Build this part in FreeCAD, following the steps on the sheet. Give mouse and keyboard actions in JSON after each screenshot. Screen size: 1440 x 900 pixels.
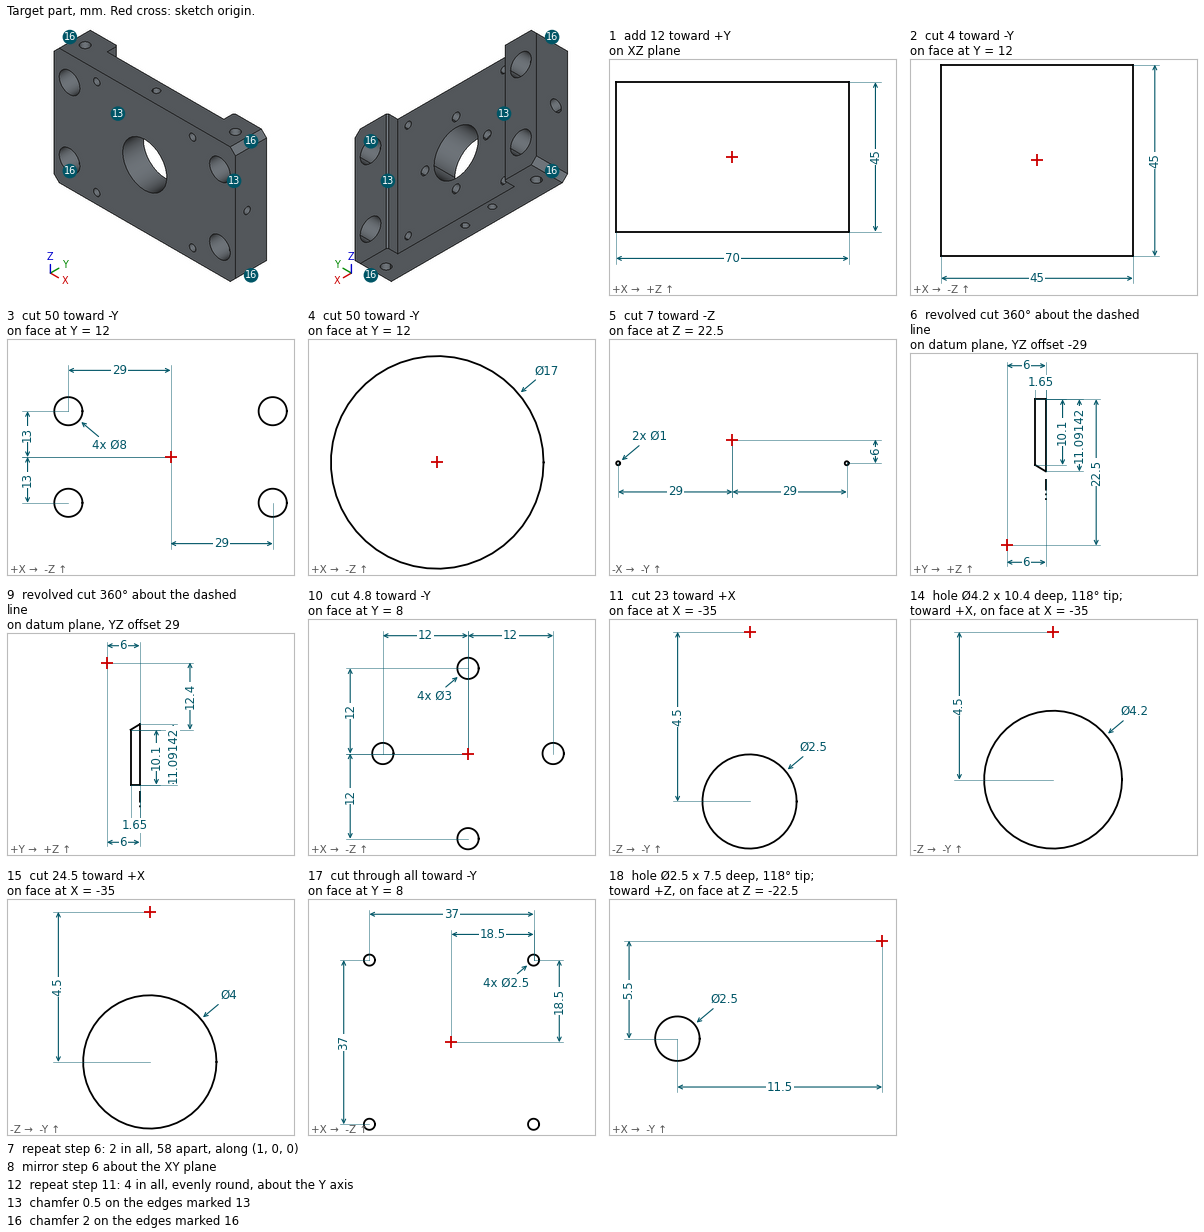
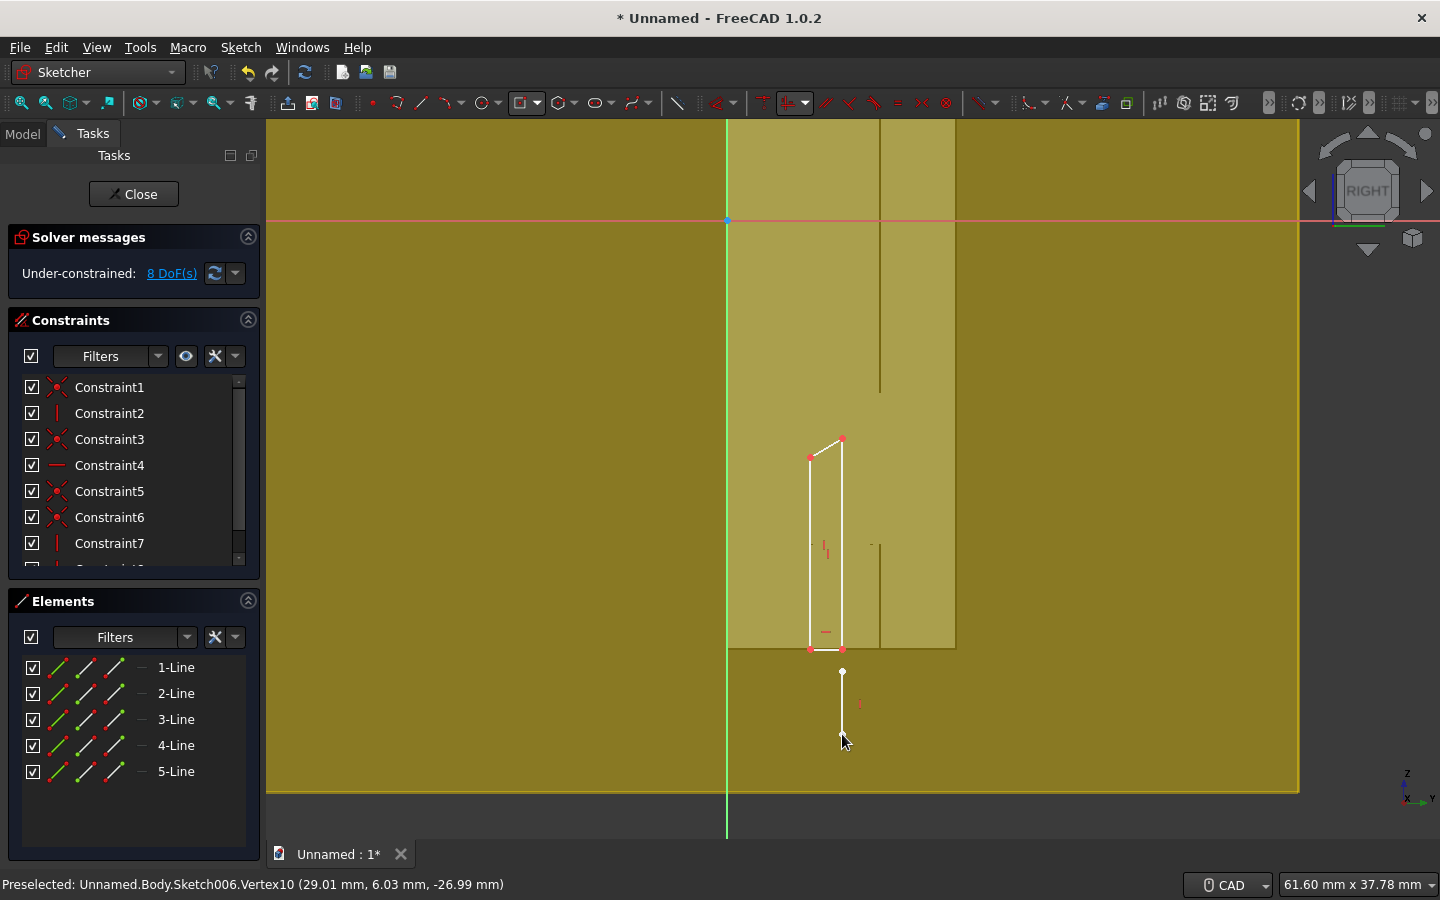
{"action": "left_click", "coordinate": [842, 691]}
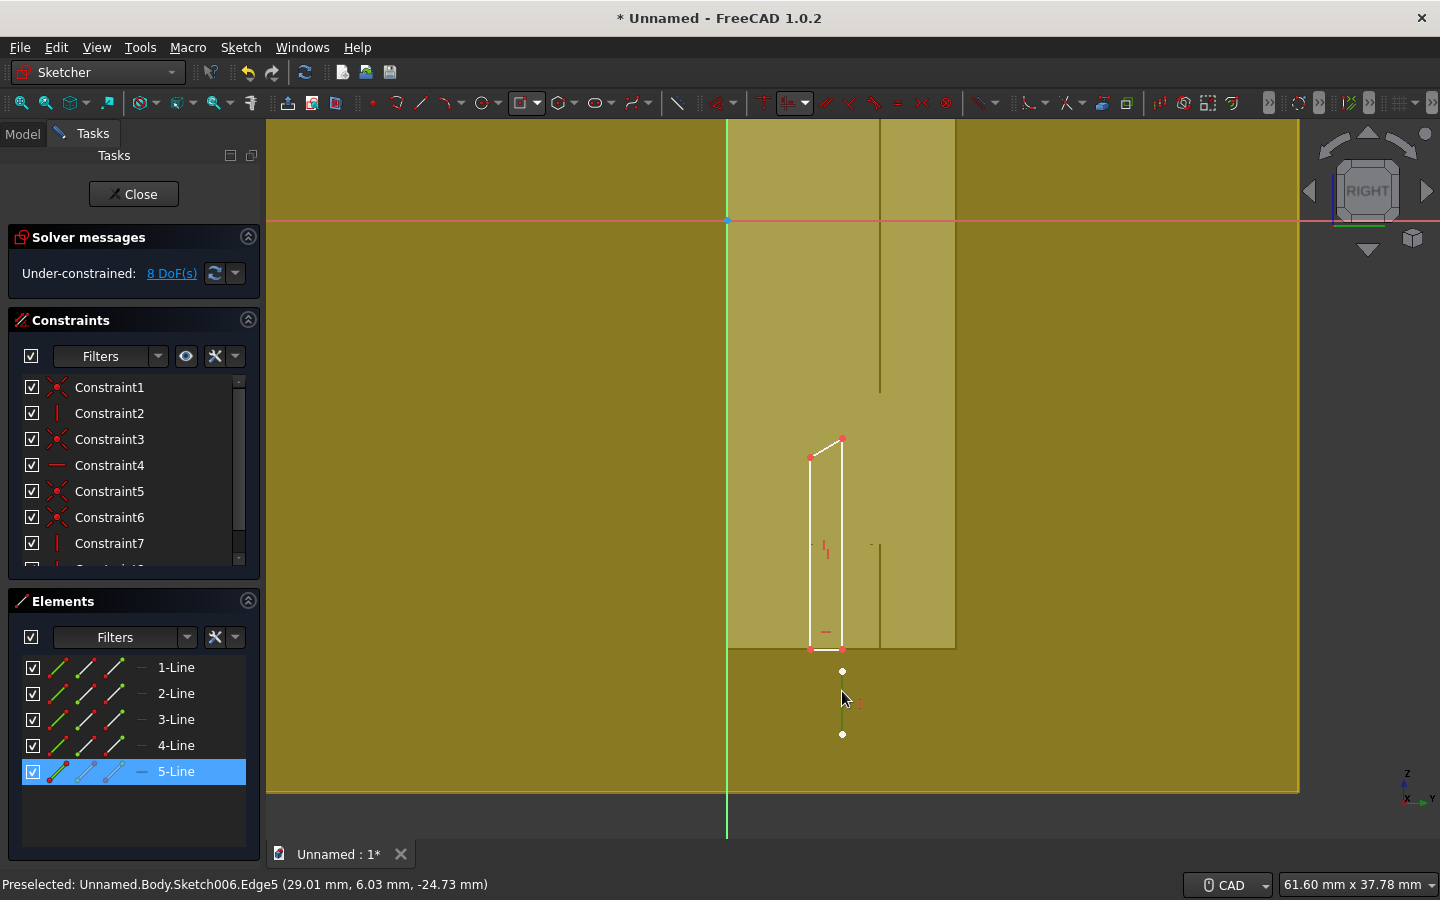
{"action": "left_click", "coordinate": [678, 104]}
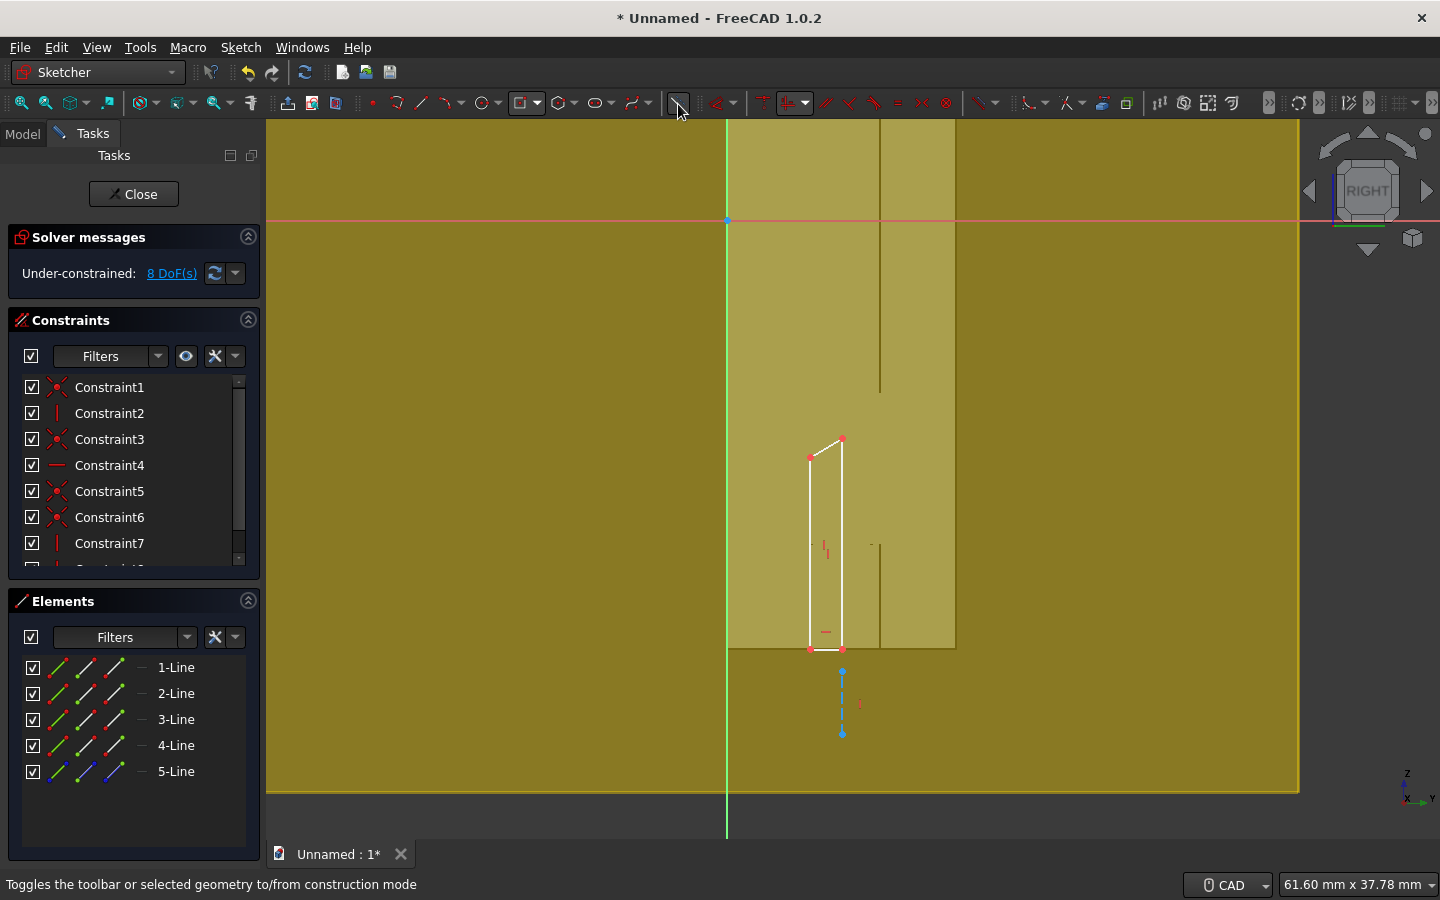
{"action": "left_click", "coordinate": [716, 104]}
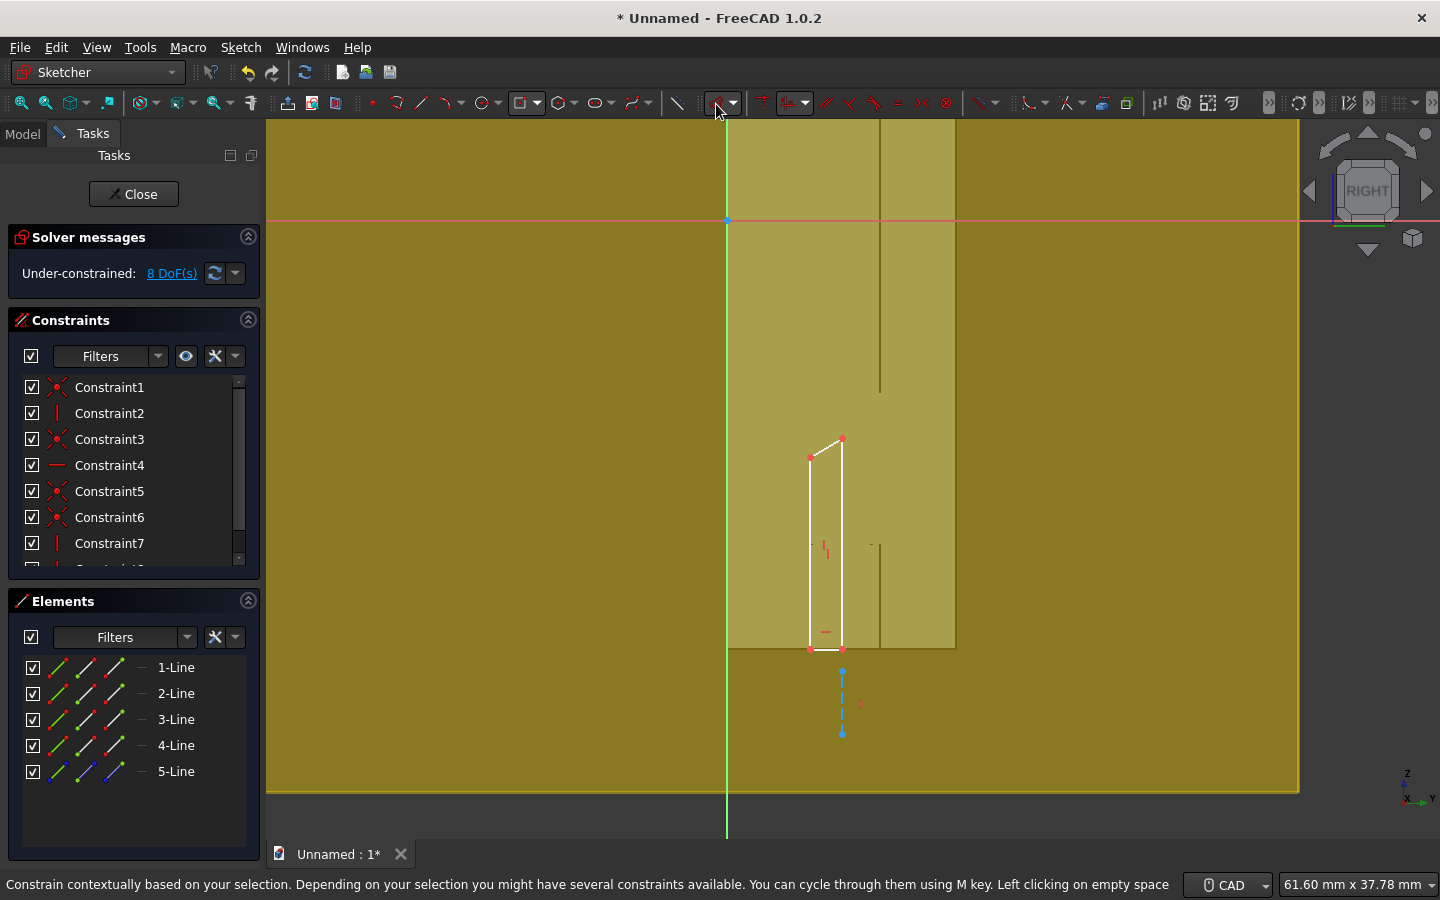
{"action": "left_click", "coordinate": [842, 439]}
{"action": "left_click", "coordinate": [785, 187]}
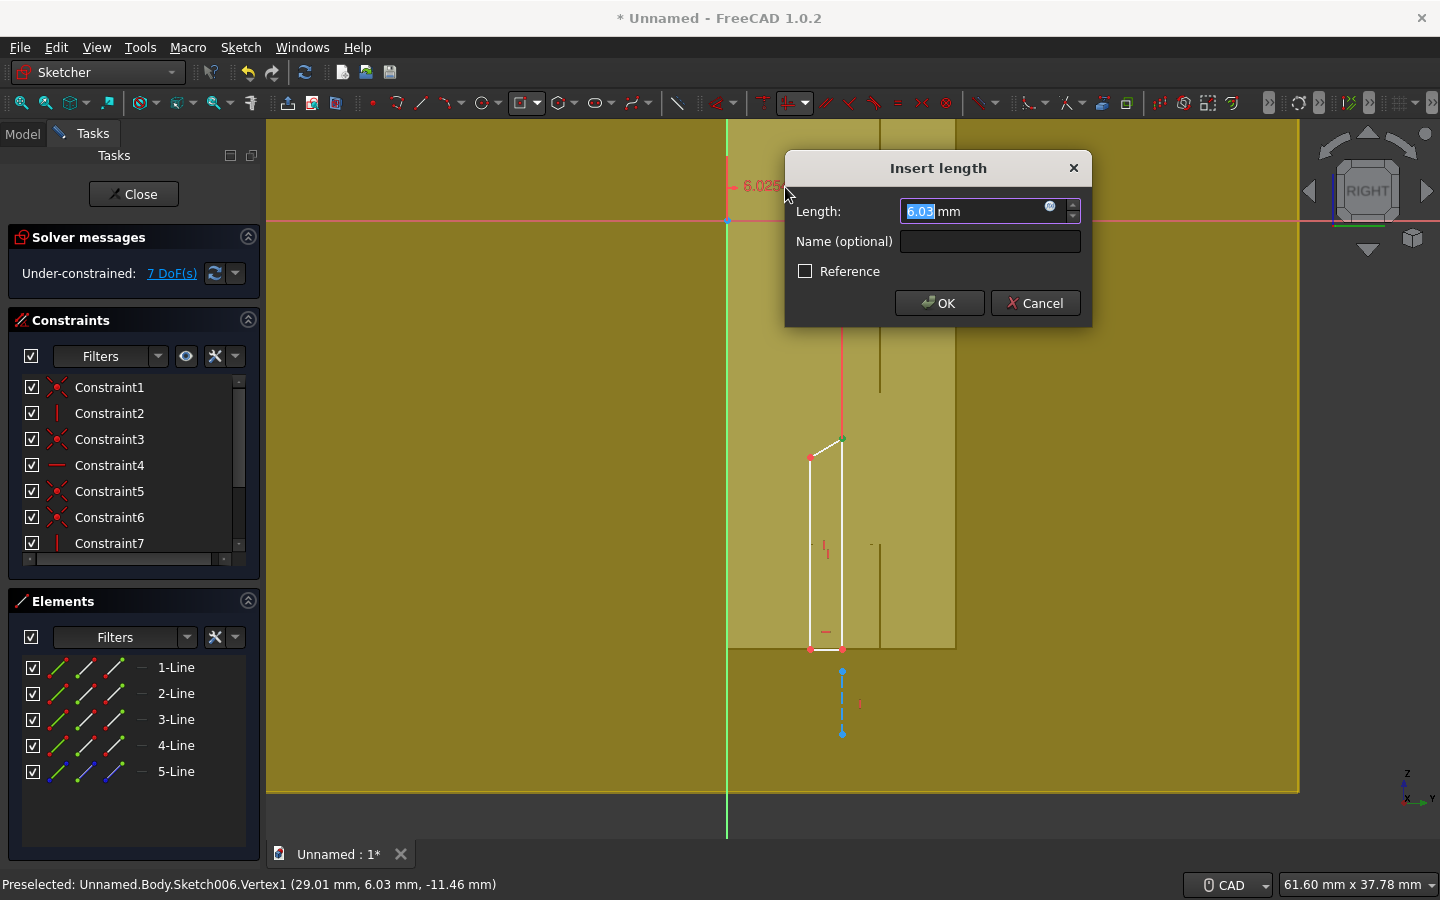
{"action": "type", "text": "6"}
{"action": "key", "text": "Return"}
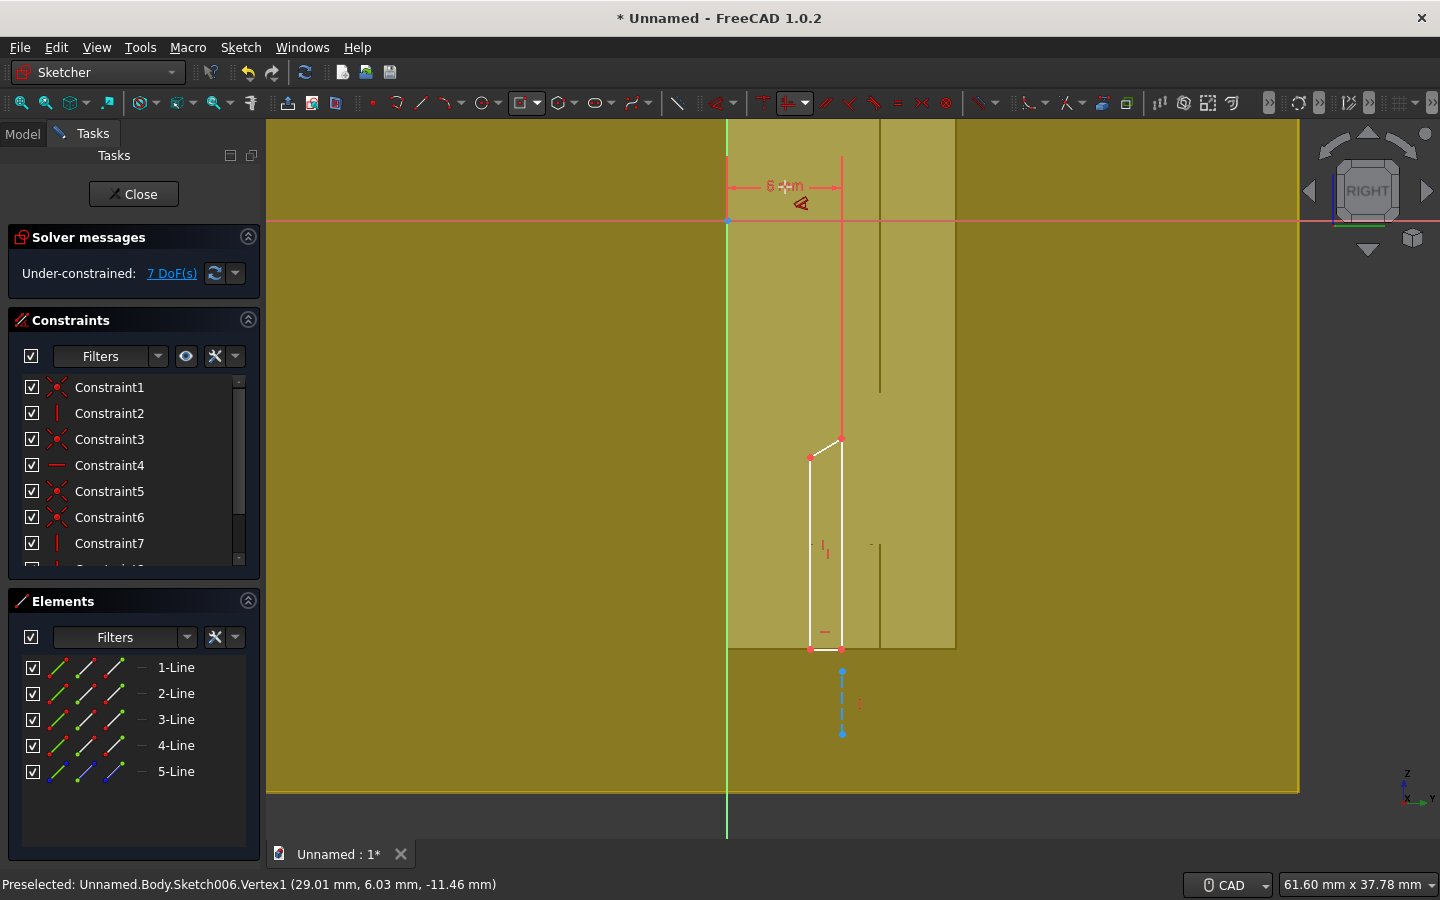
{"action": "left_click", "coordinate": [842, 672]}
{"action": "left_click", "coordinate": [785, 706]}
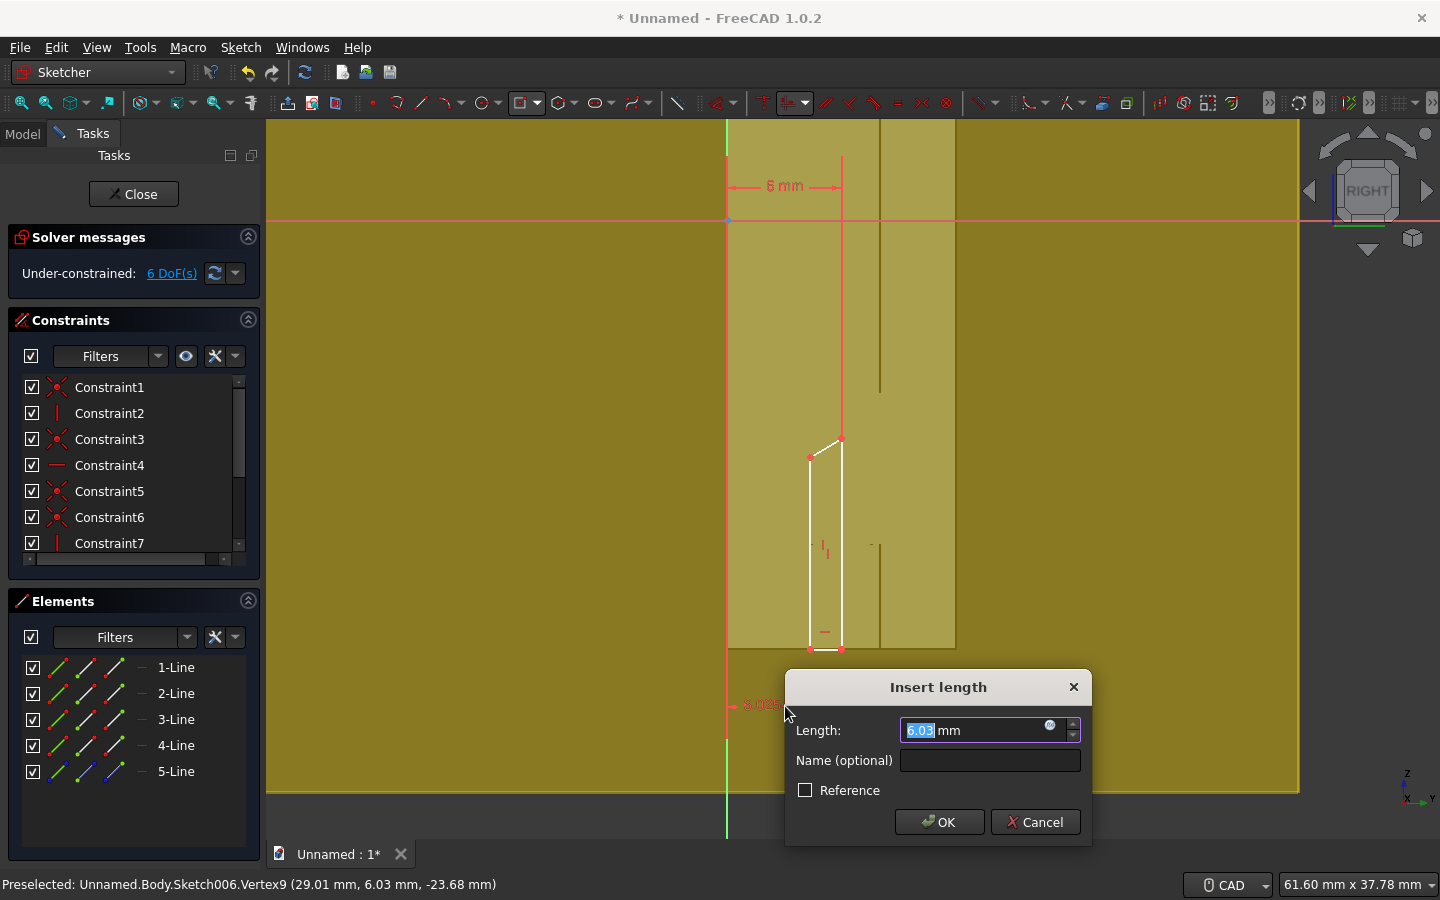
{"action": "type", "text": "6"}
{"action": "key", "text": "Return"}